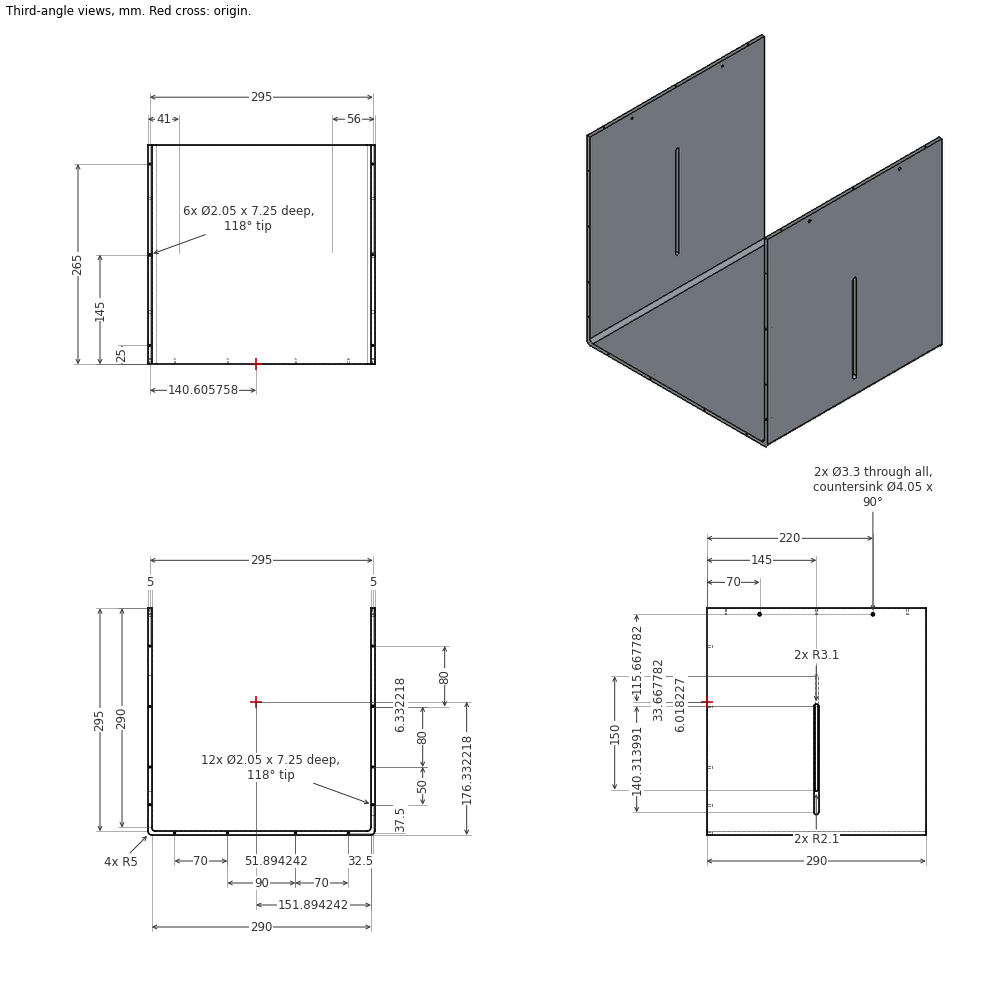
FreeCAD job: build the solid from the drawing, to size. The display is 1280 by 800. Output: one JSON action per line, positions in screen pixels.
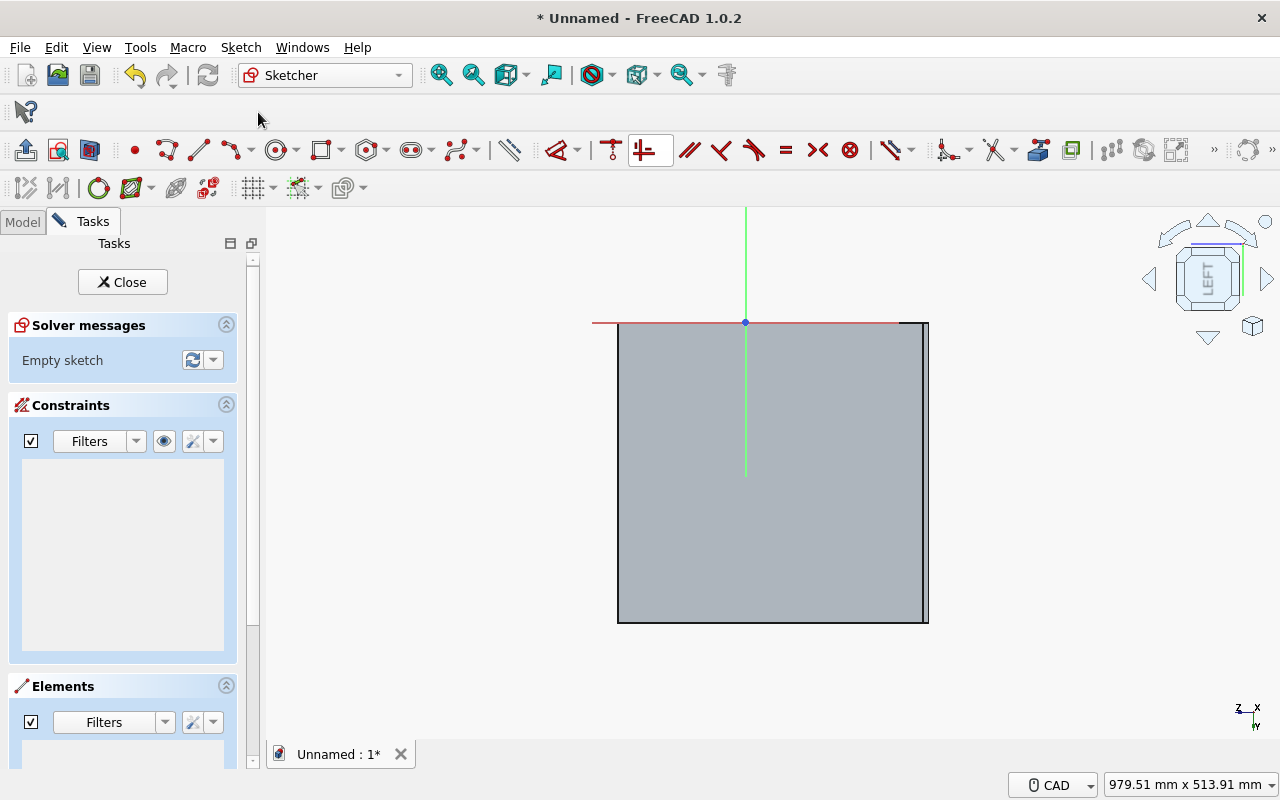
{"action": "scroll", "coordinate": [857, 339], "scroll_direction": "up", "scroll_amount": 4}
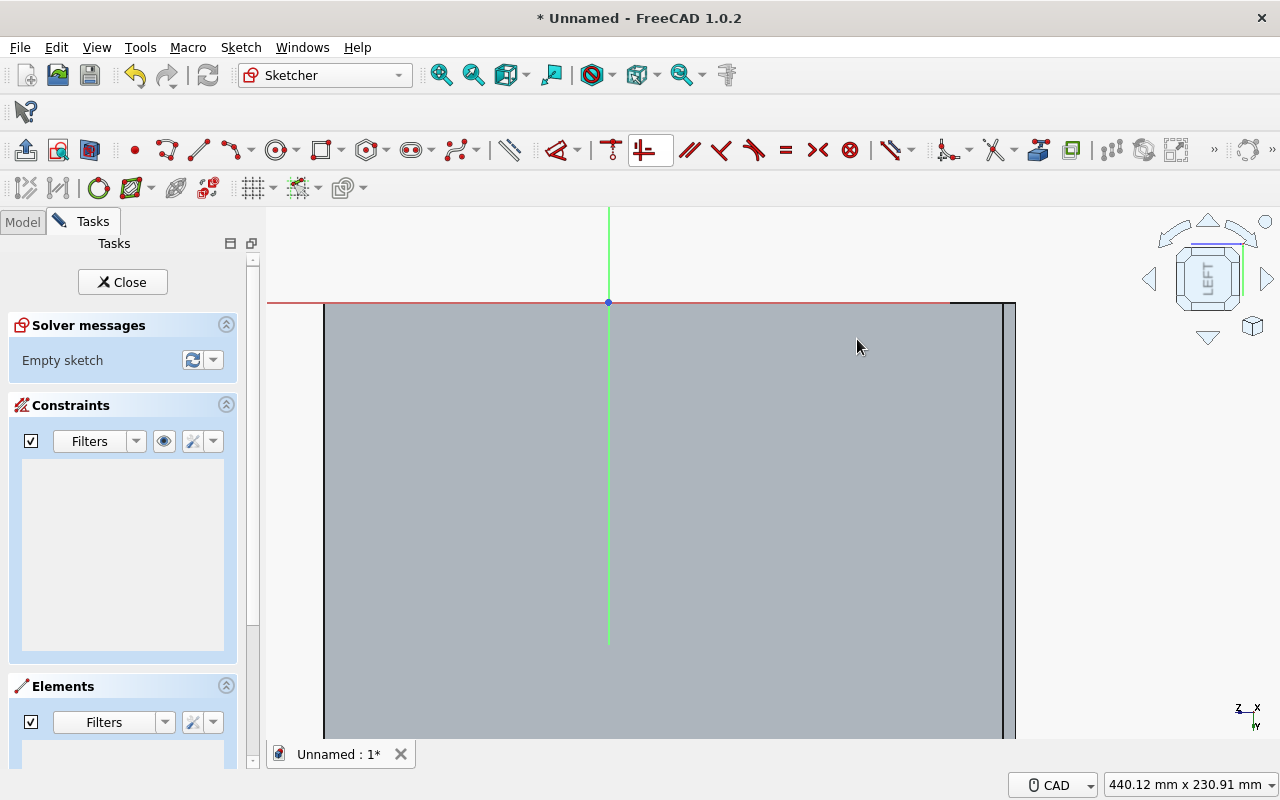
{"action": "left_click", "coordinate": [412, 150]}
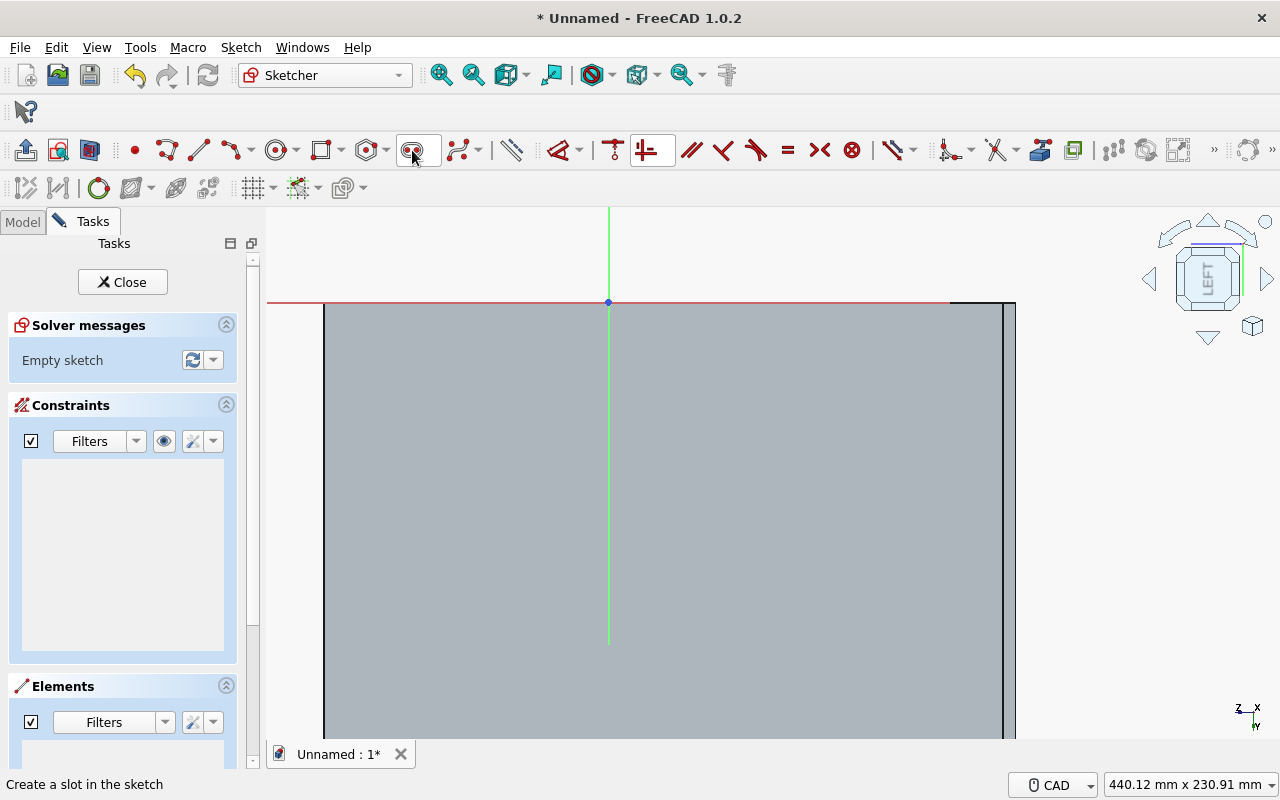
{"action": "scroll", "coordinate": [531, 637], "scroll_direction": "up", "scroll_amount": 8}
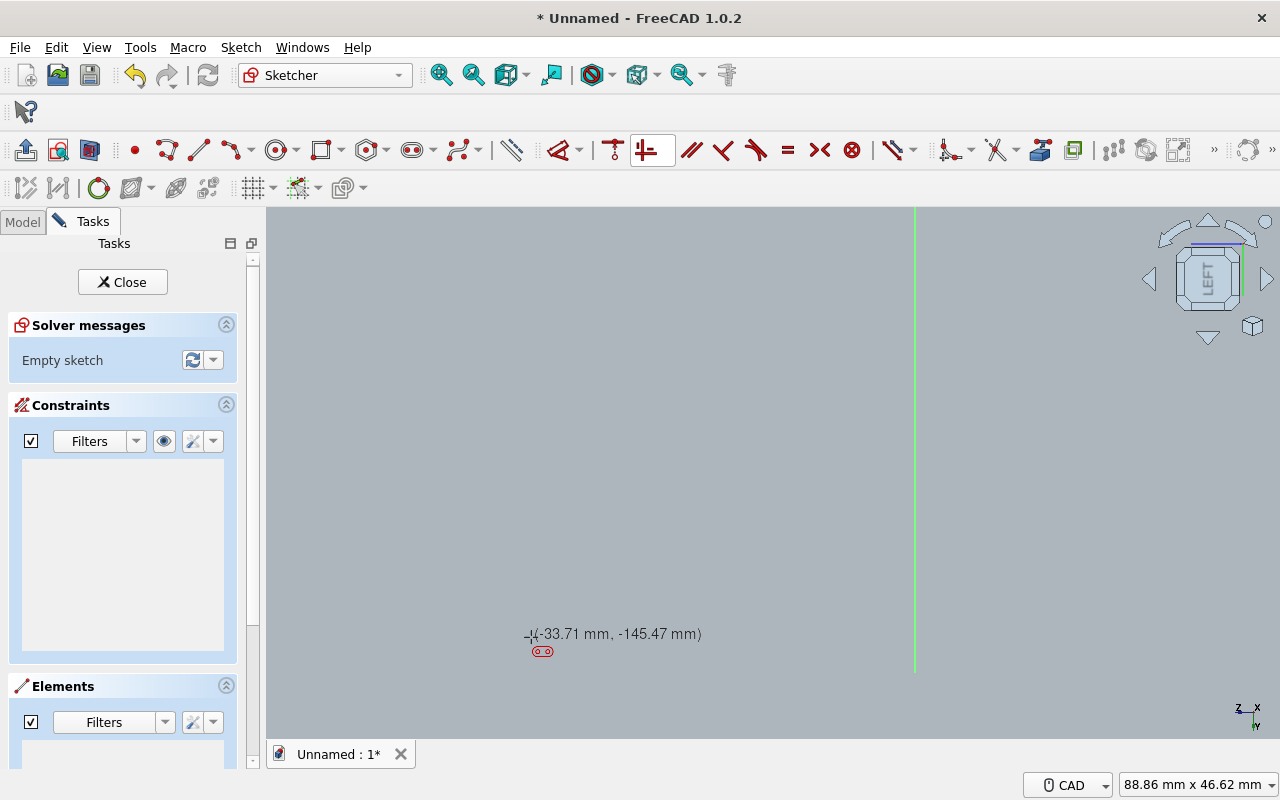
{"action": "scroll", "coordinate": [532, 639], "scroll_direction": "down", "scroll_amount": 8}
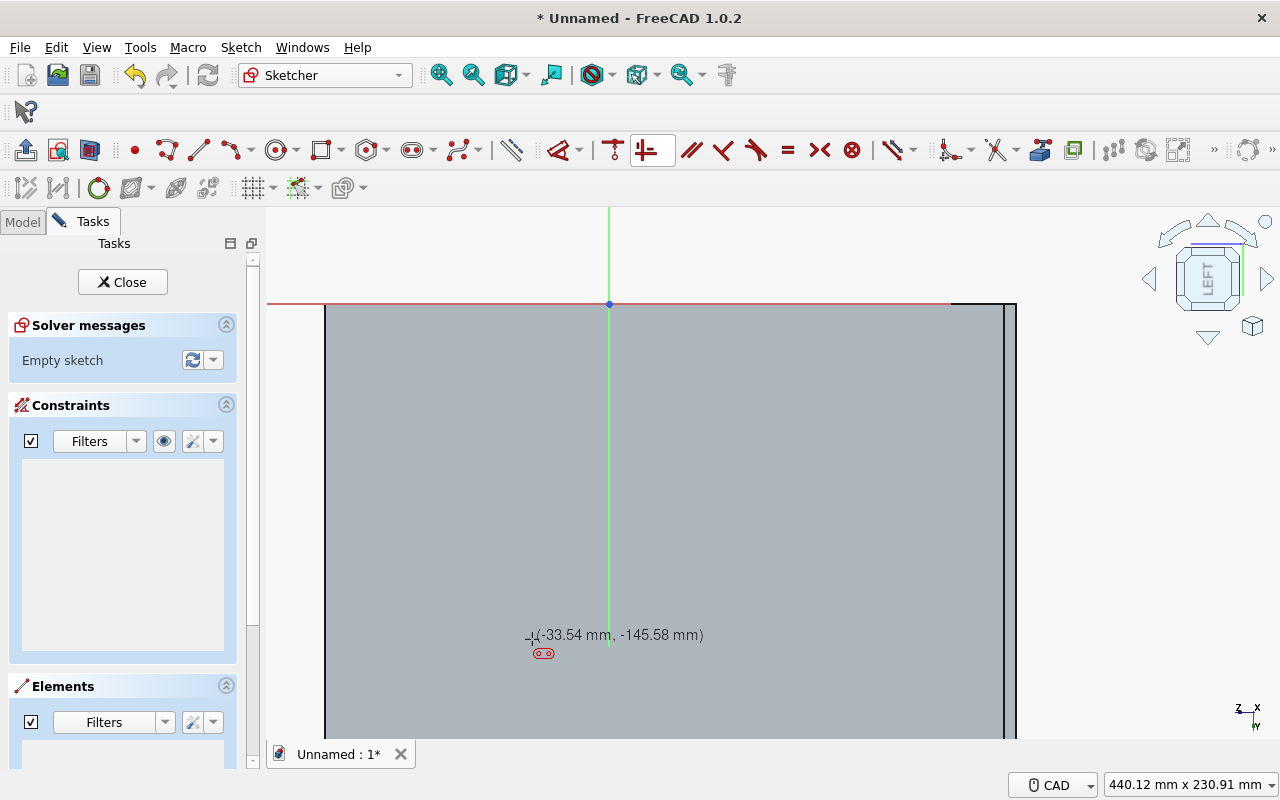
{"action": "left_click", "coordinate": [532, 639]}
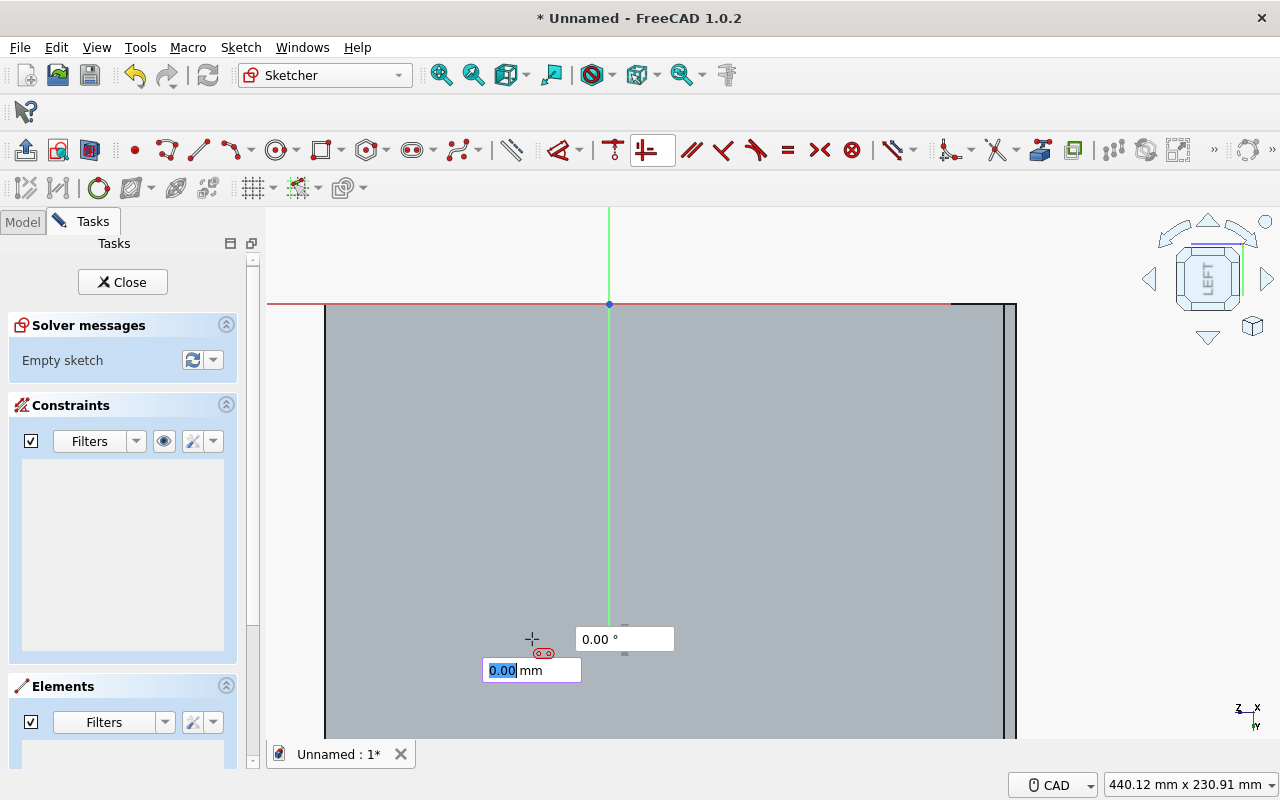
{"action": "left_click", "coordinate": [877, 639]}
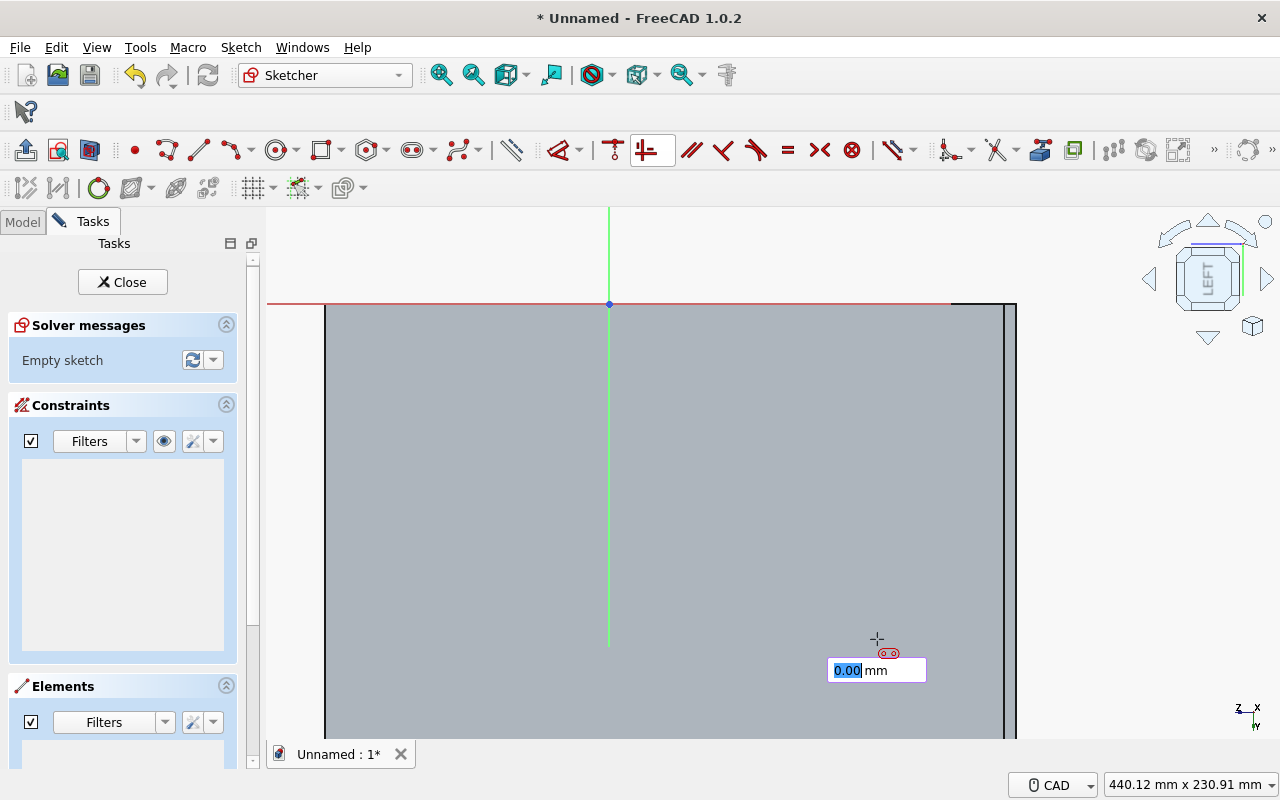
{"action": "scroll", "coordinate": [705, 643], "scroll_direction": "up", "scroll_amount": 6}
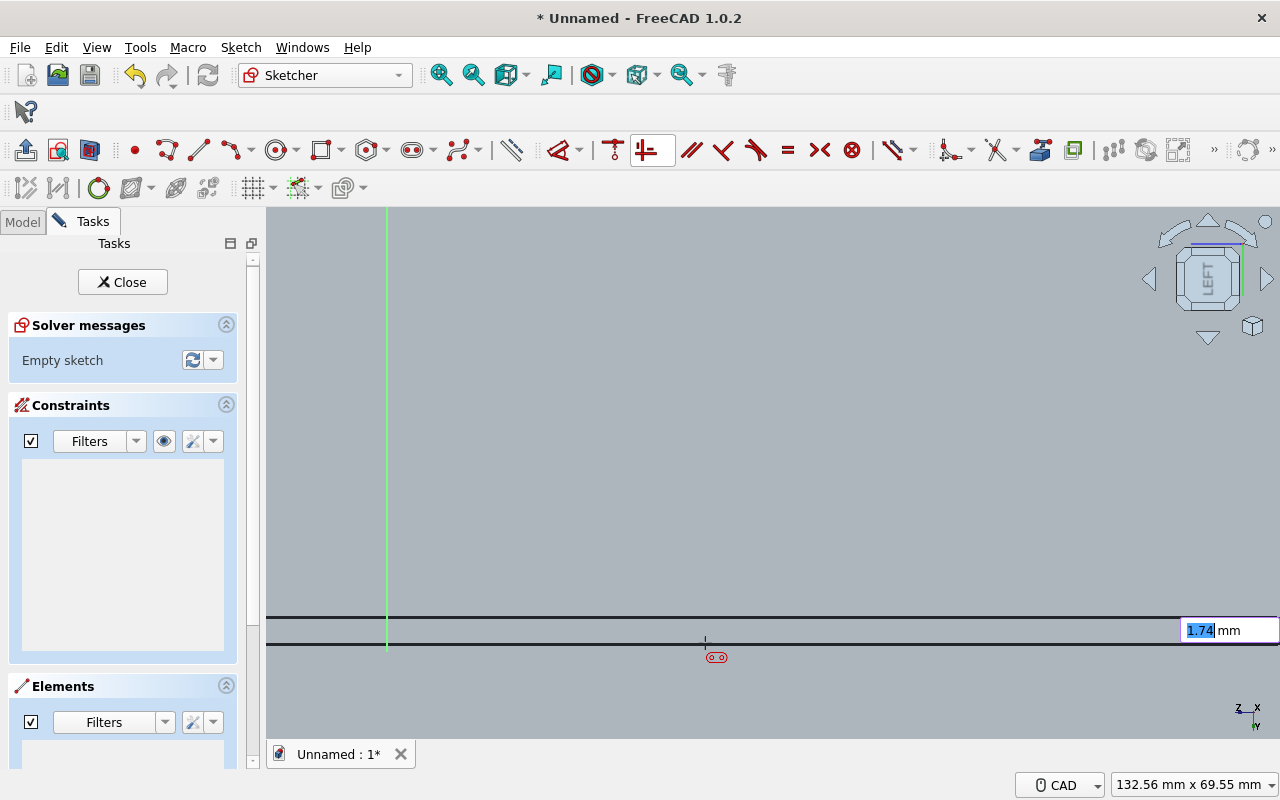
{"action": "left_click", "coordinate": [703, 642]}
{"action": "key", "text": "Escape"}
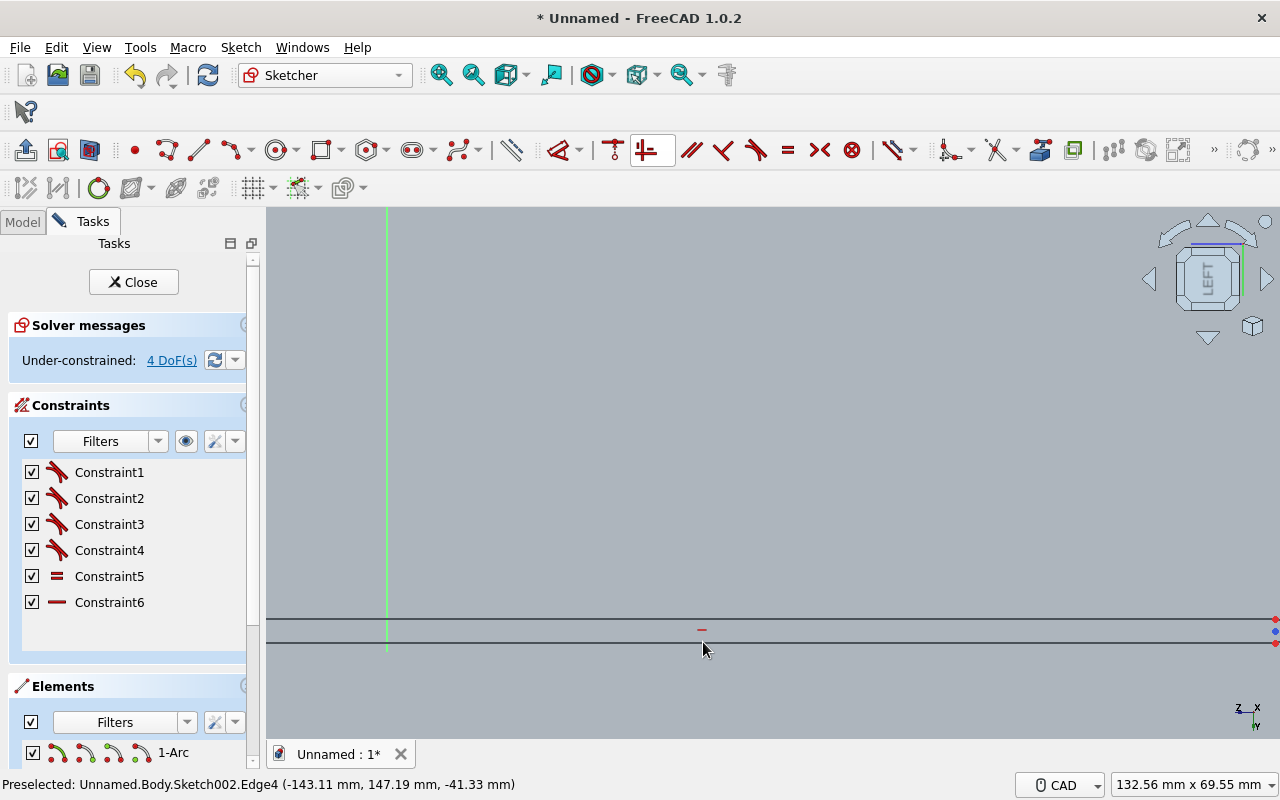
{"action": "left_click", "coordinate": [558, 150]}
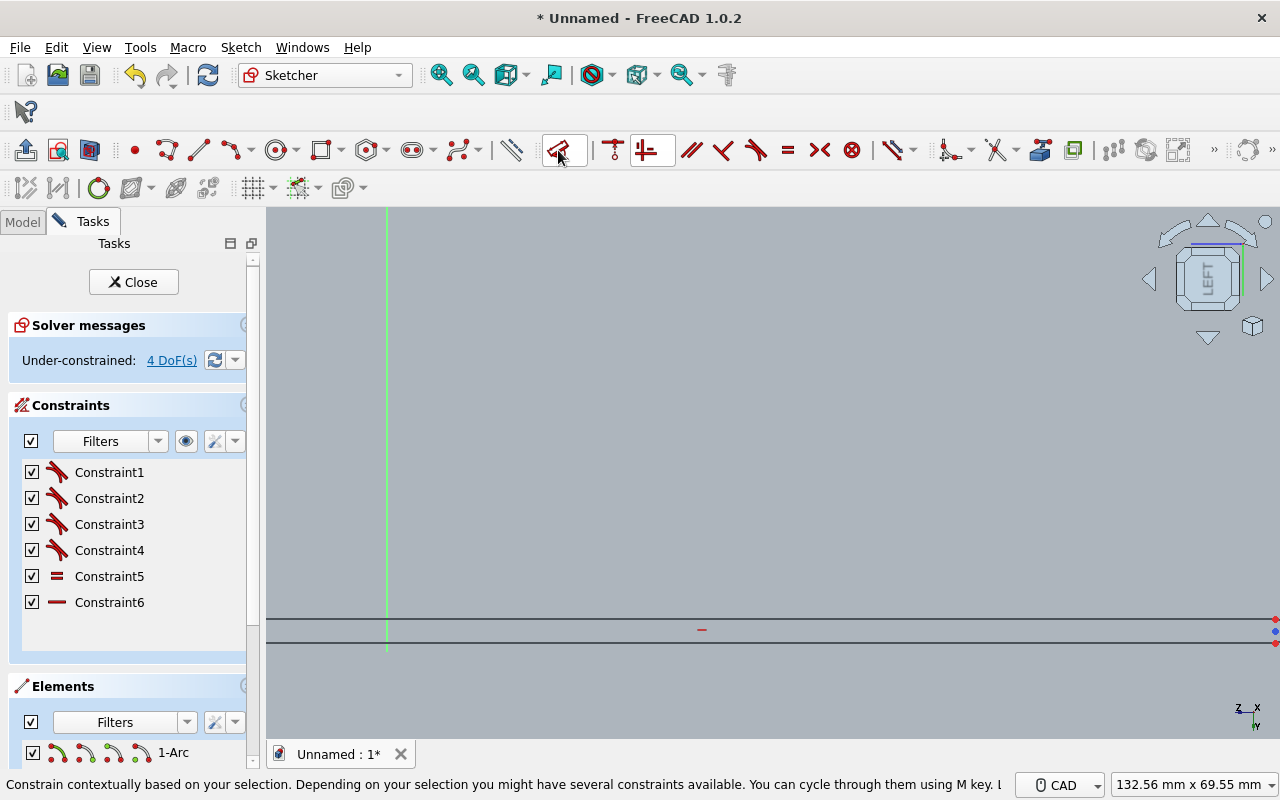
{"action": "scroll", "coordinate": [705, 643], "scroll_direction": "down", "scroll_amount": 6}